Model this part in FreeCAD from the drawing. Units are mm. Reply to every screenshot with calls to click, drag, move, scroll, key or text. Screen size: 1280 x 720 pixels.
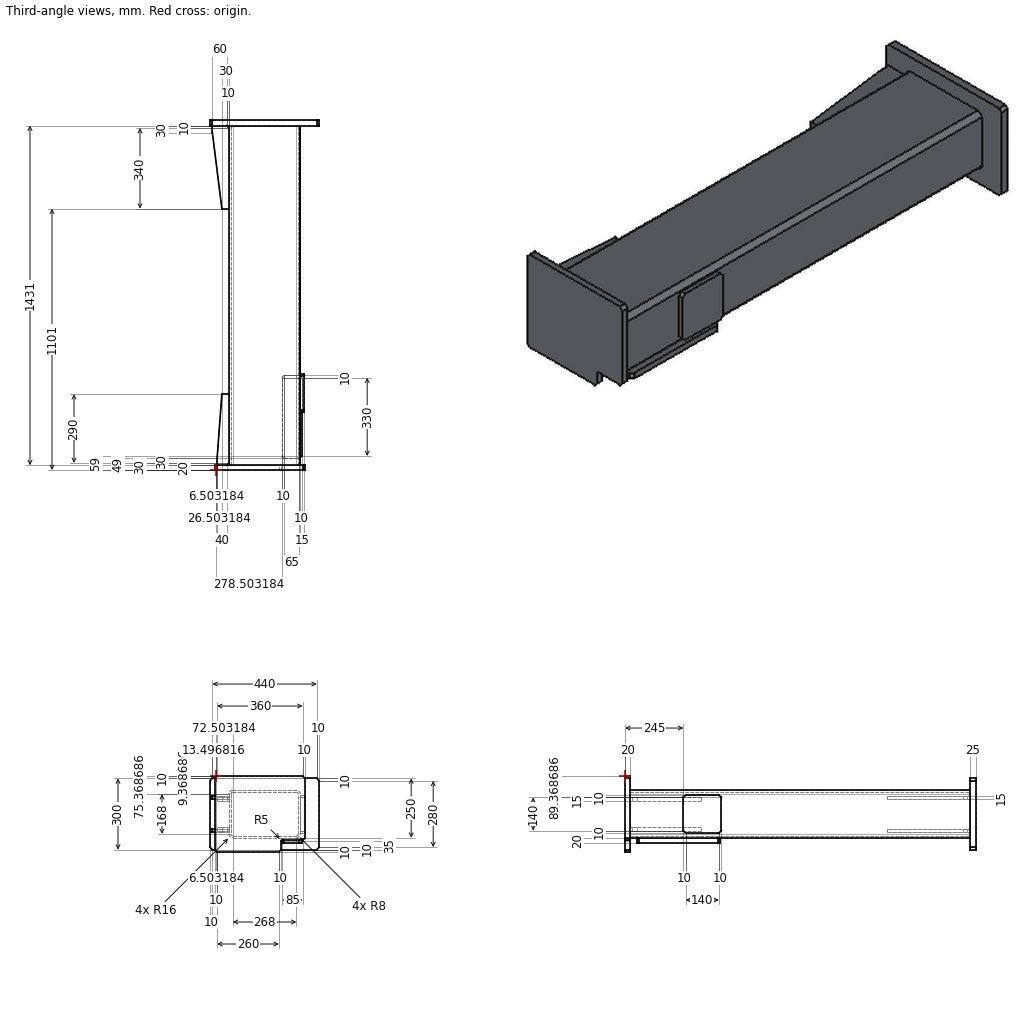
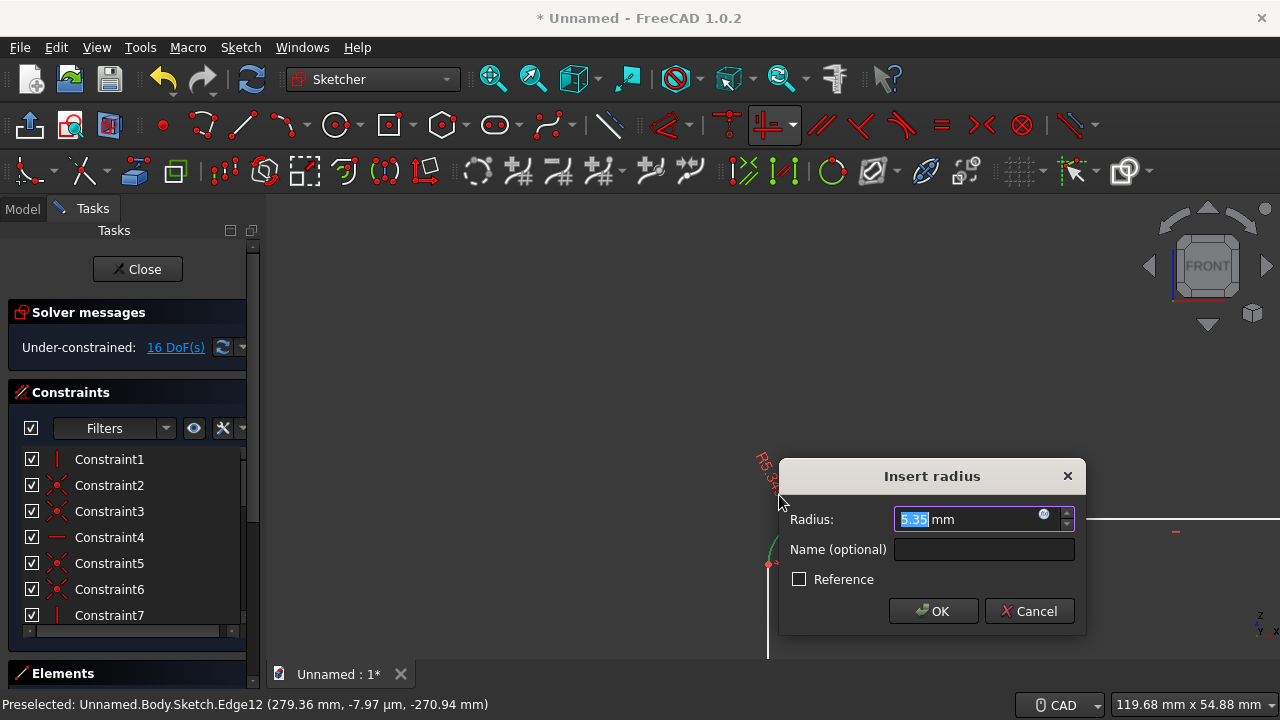
text(5)
key(Return)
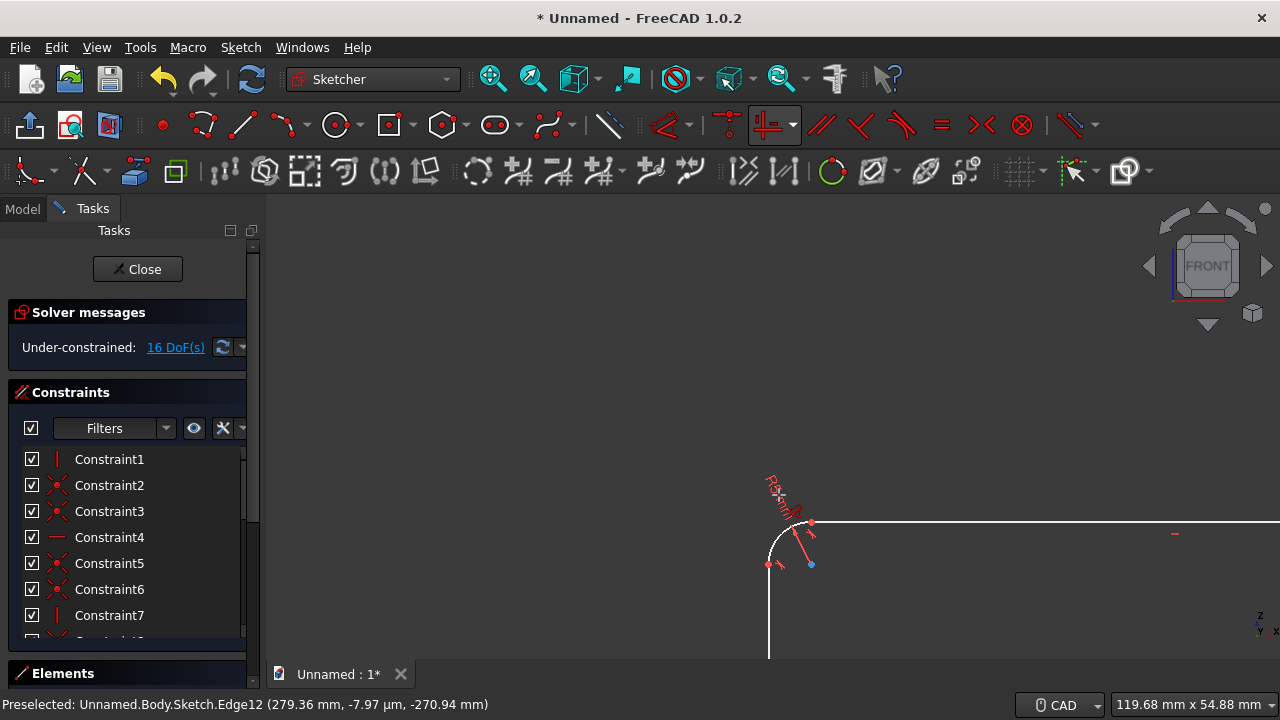
scroll(791, 532, down, 11)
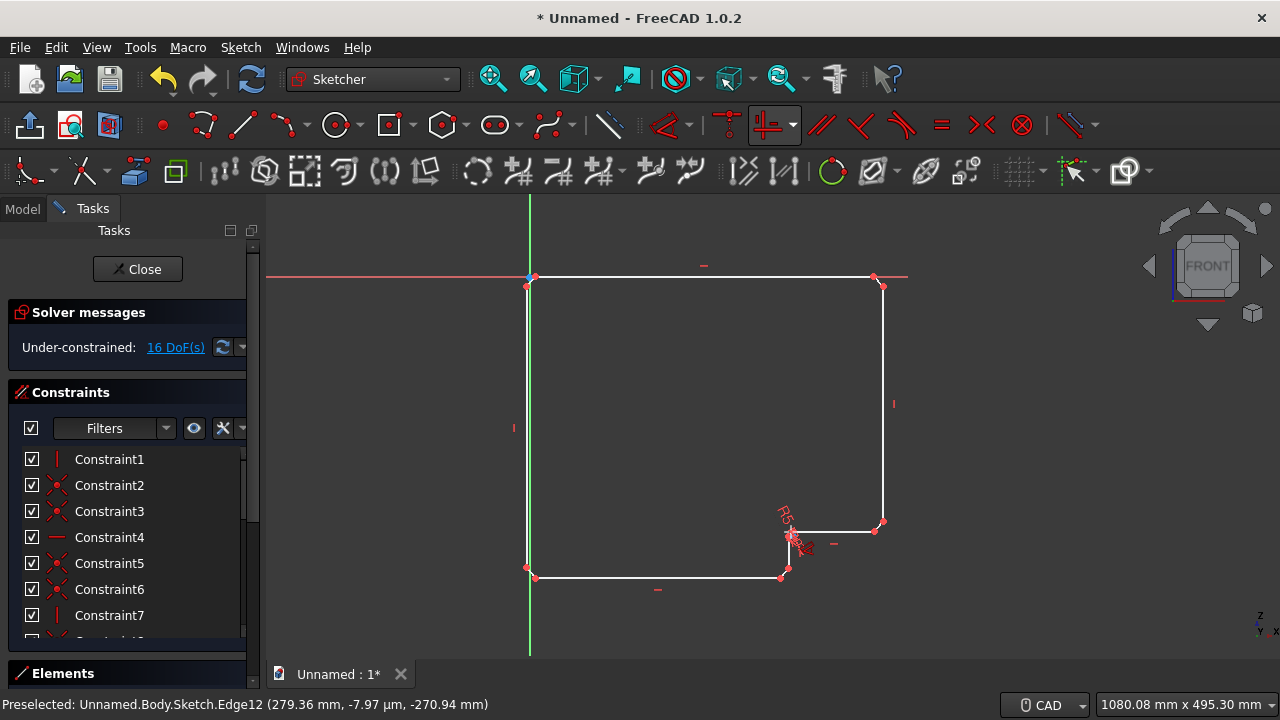
scroll(789, 543, up, 4)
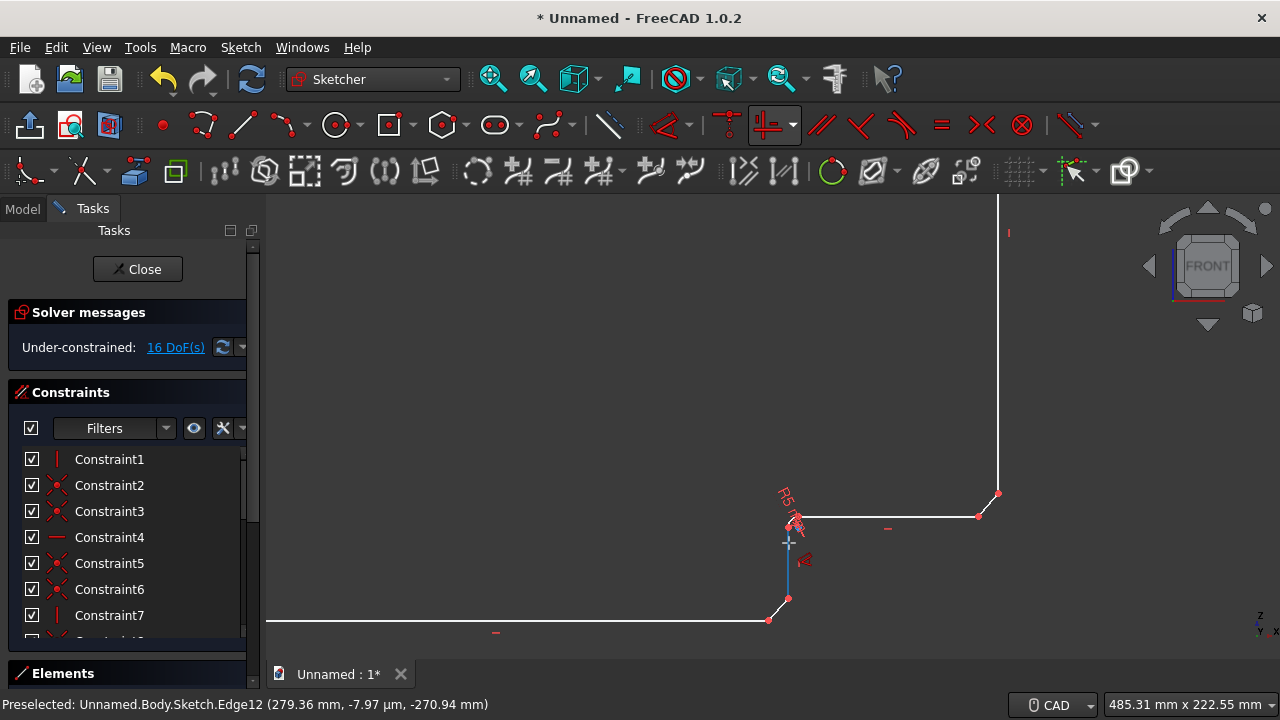
click(788, 541)
click(822, 563)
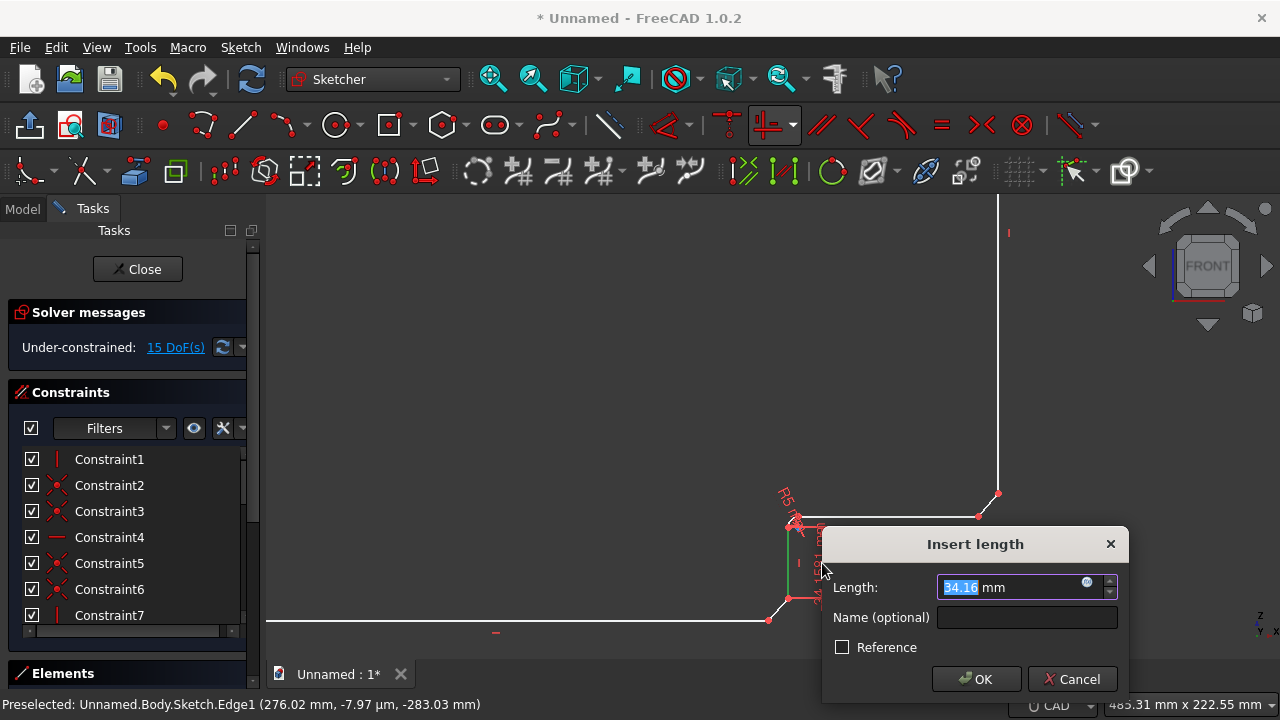
text(35)
key(Return)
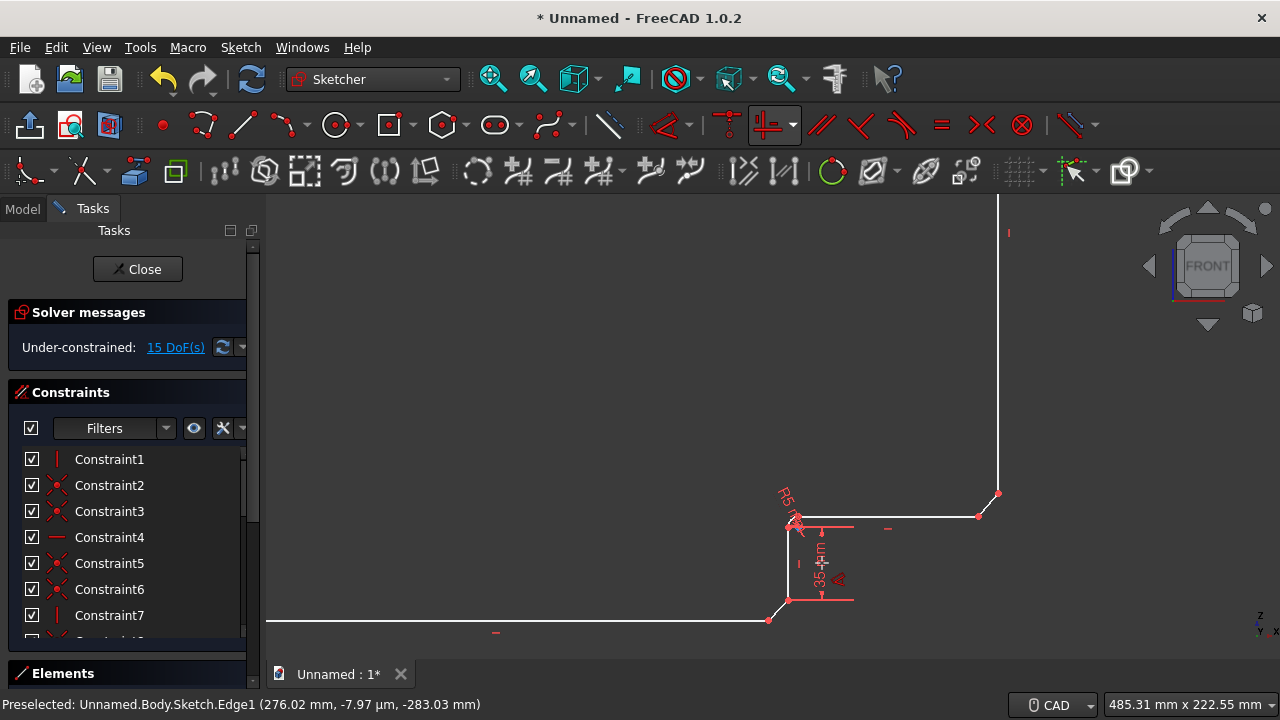
click(924, 517)
click(930, 551)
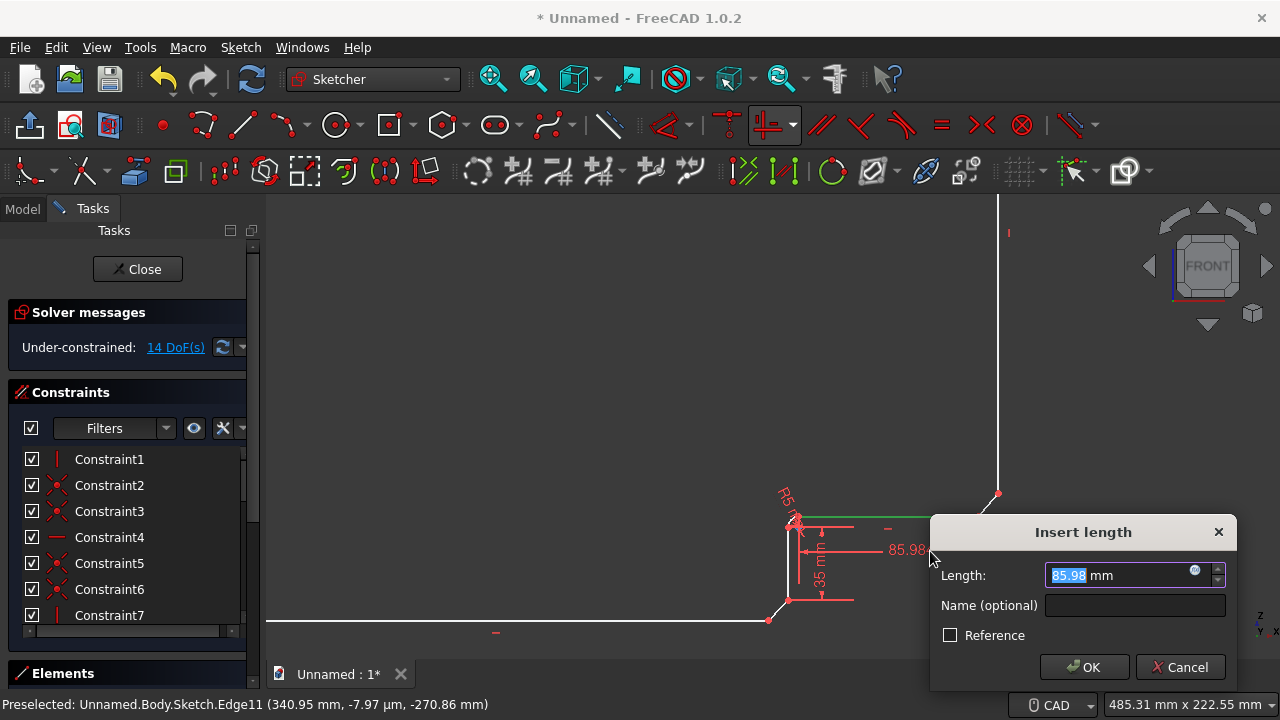
text(85)
key(Return)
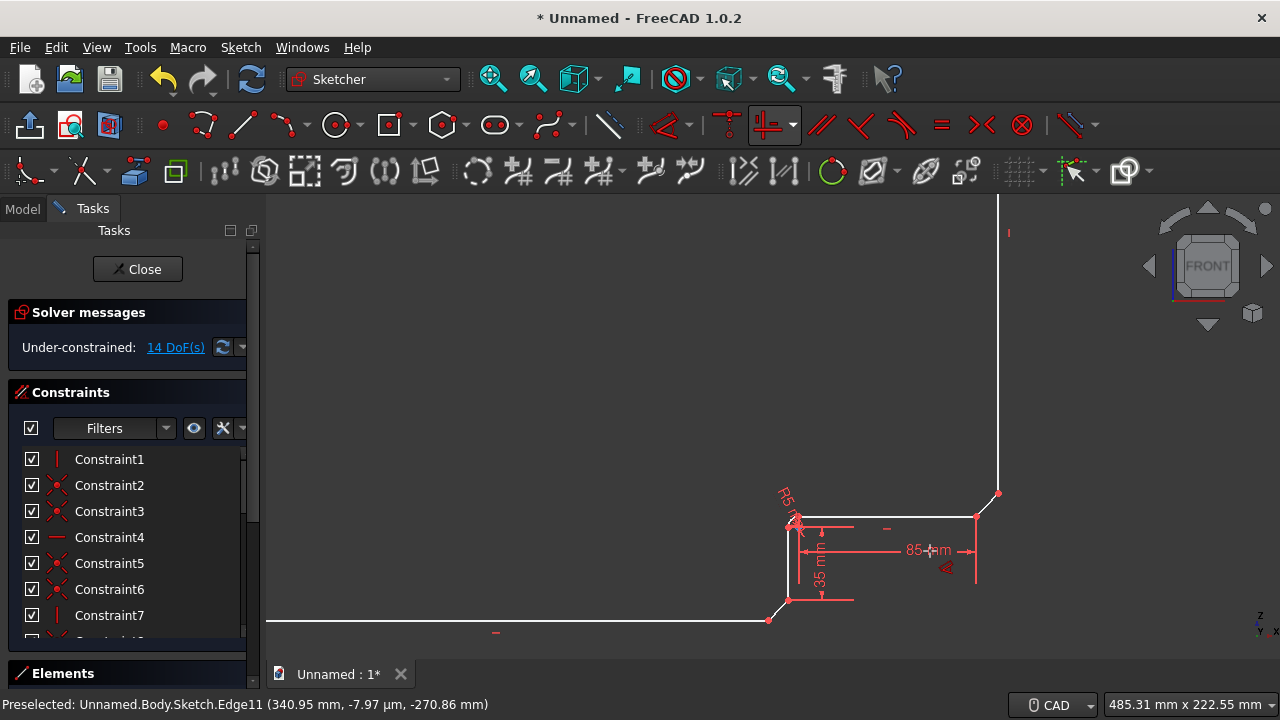
click(606, 621)
click(531, 587)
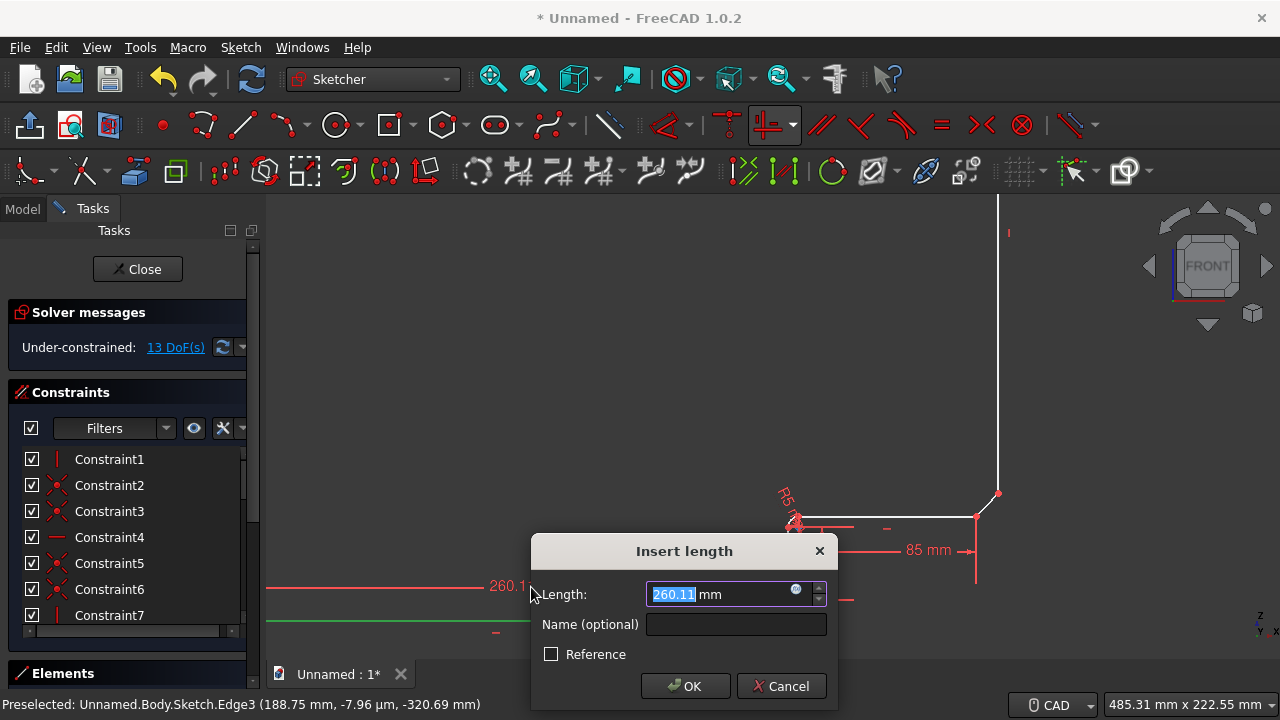
text(260)
key(Return)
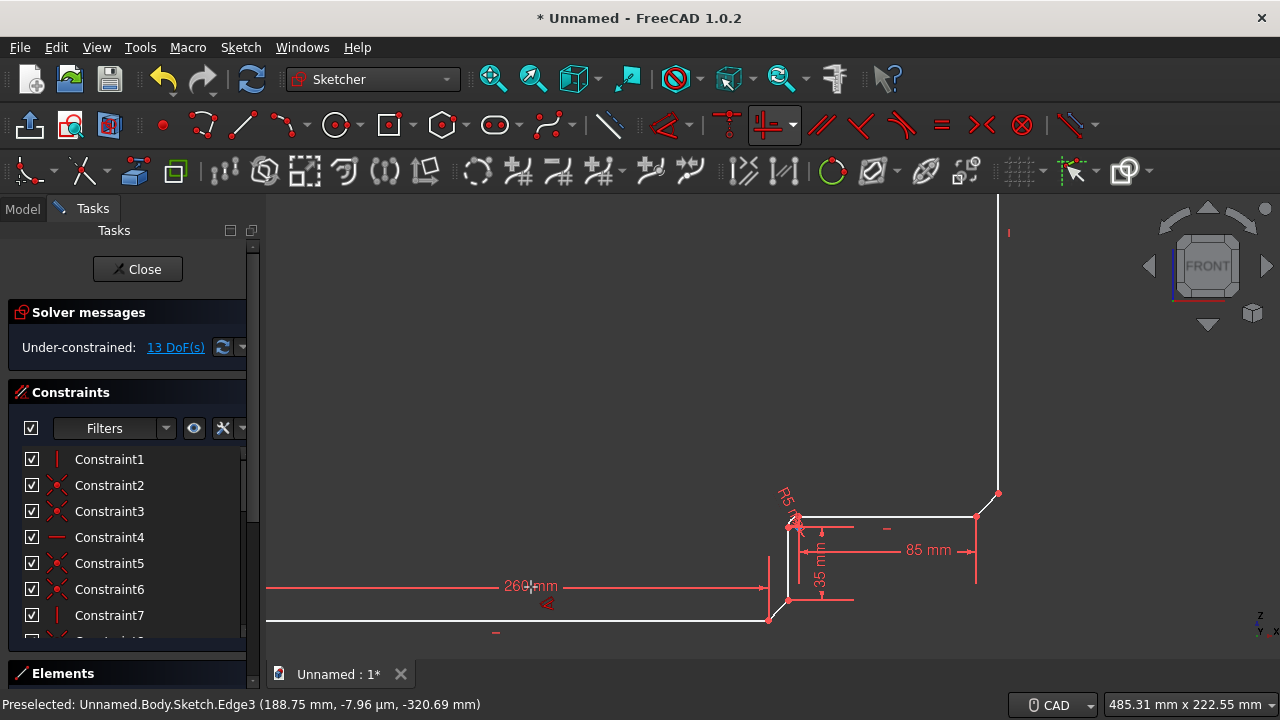
scroll(789, 543, down, 4)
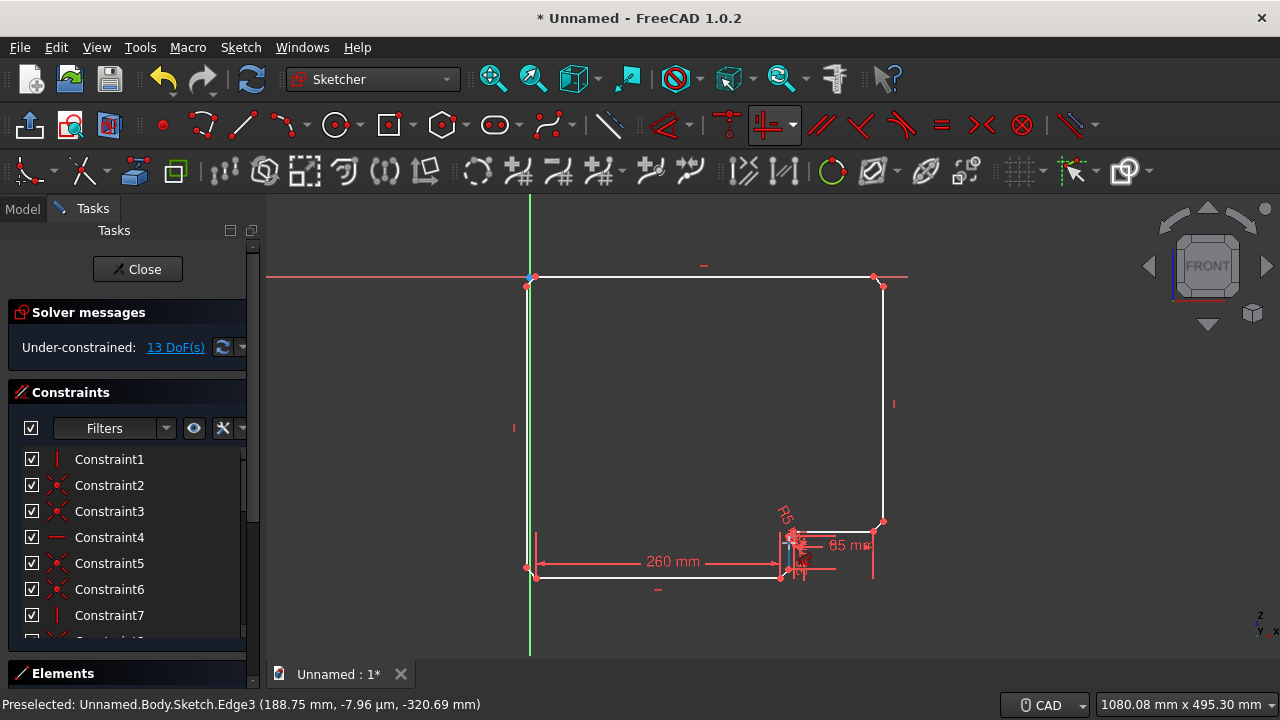
scroll(527, 483, up, 8)